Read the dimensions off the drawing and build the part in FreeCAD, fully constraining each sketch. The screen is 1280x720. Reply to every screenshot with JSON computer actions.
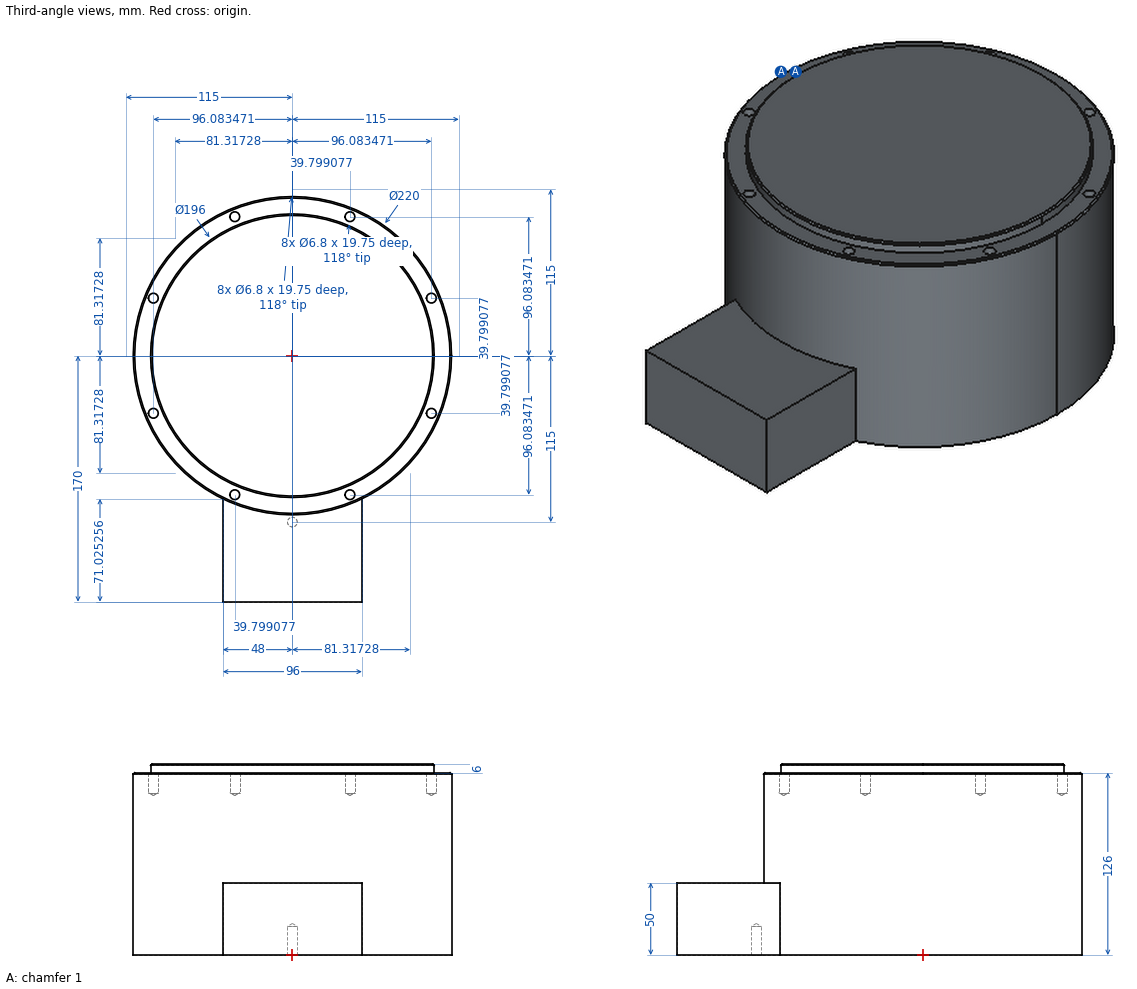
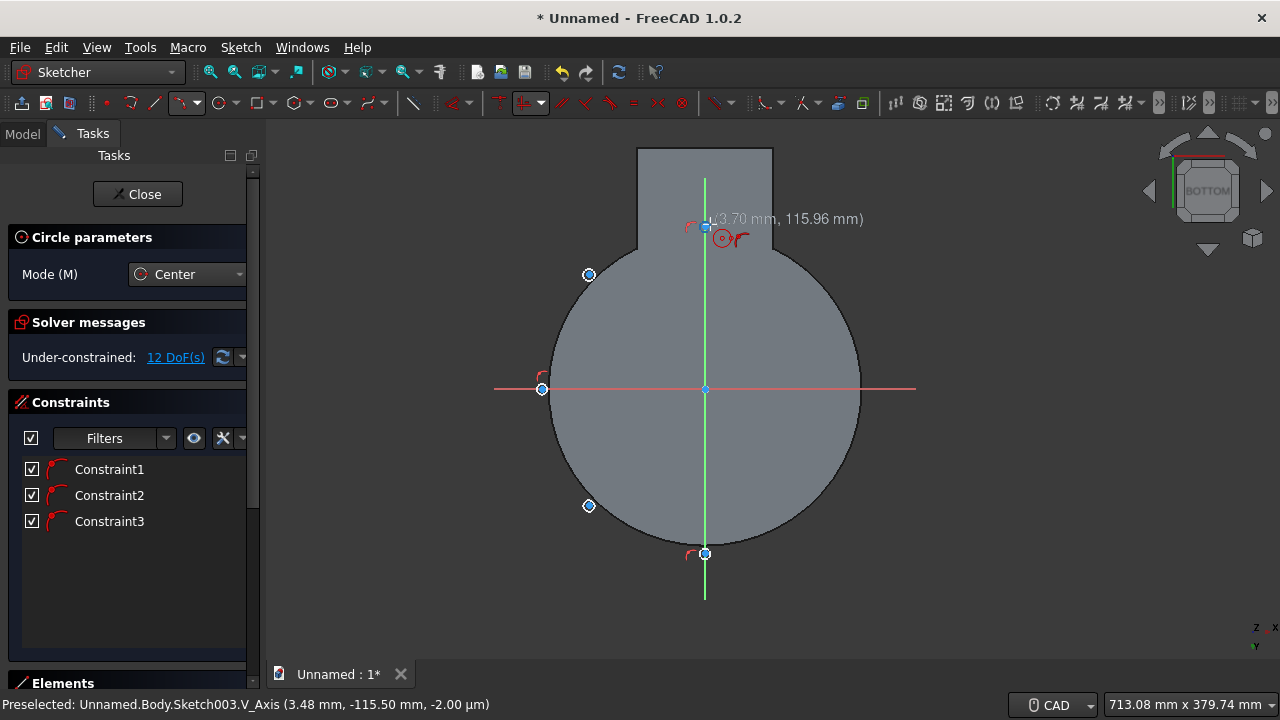
{"action": "scroll", "coordinate": [821, 274], "scroll_direction": "up", "scroll_amount": 8}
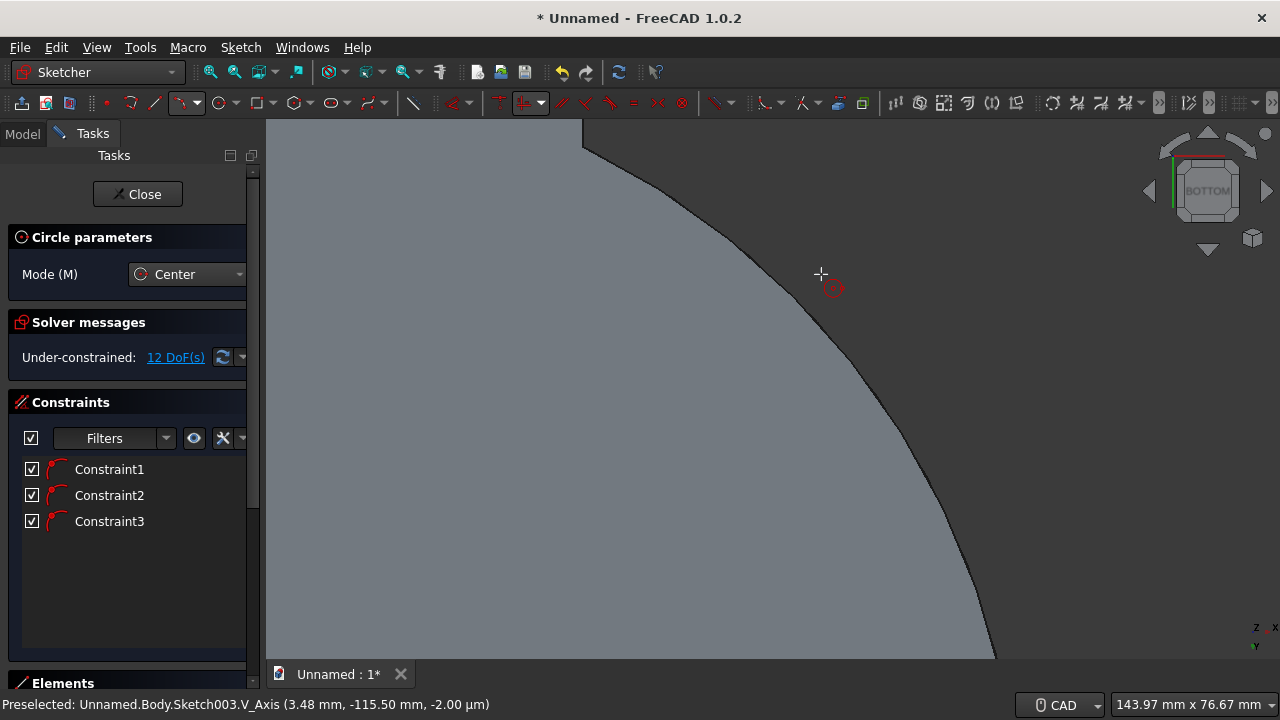
{"action": "scroll", "coordinate": [821, 274], "scroll_direction": "down", "scroll_amount": 8}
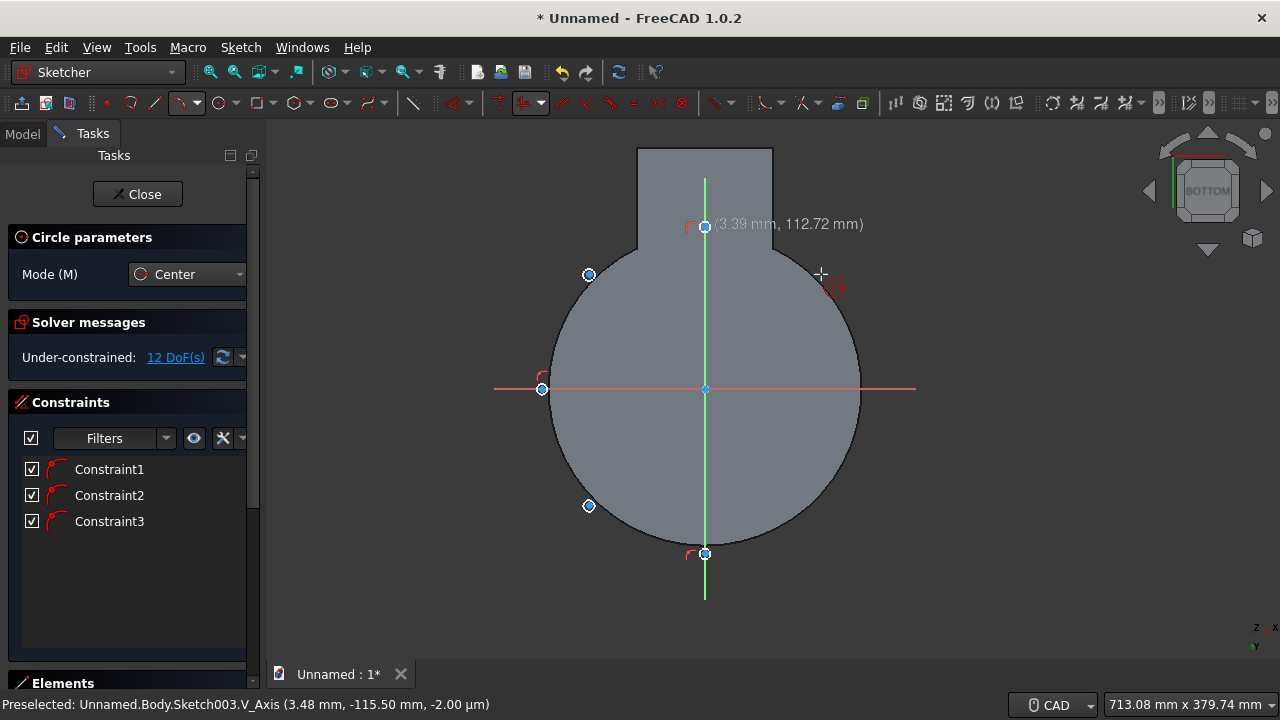
{"action": "left_click", "coordinate": [821, 274]}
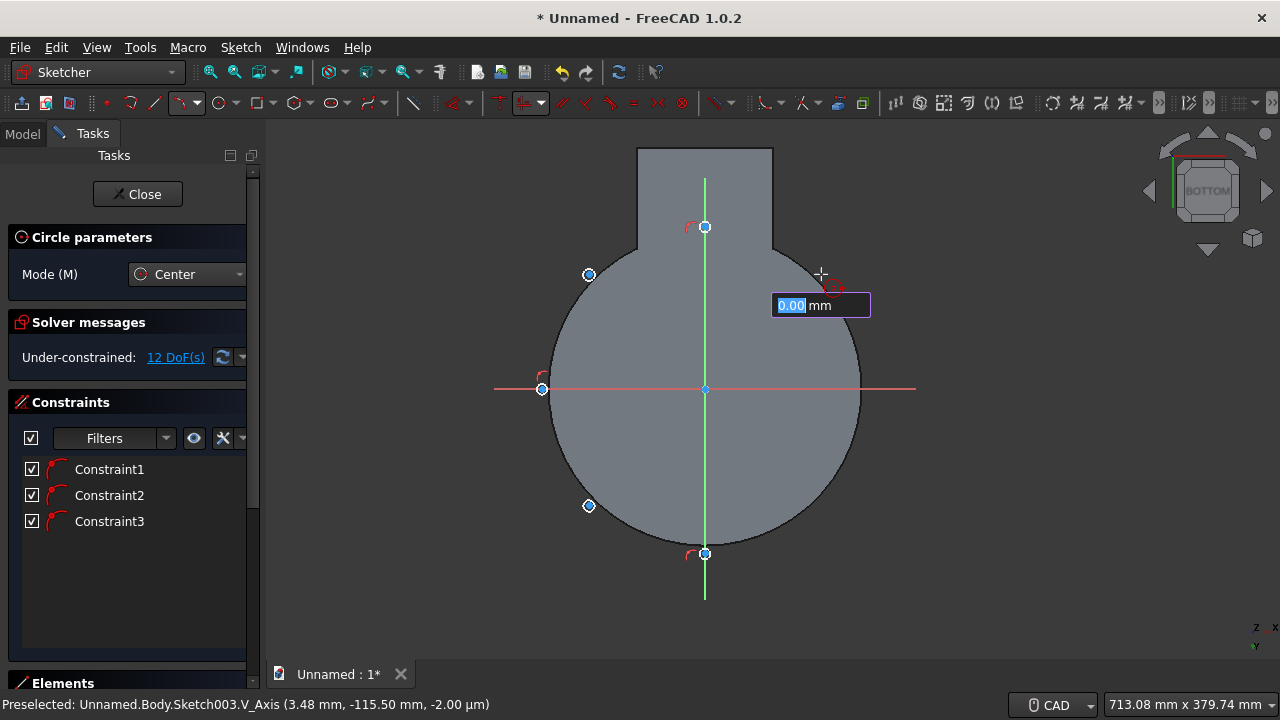
{"action": "scroll", "coordinate": [824, 270], "scroll_direction": "up", "scroll_amount": 6}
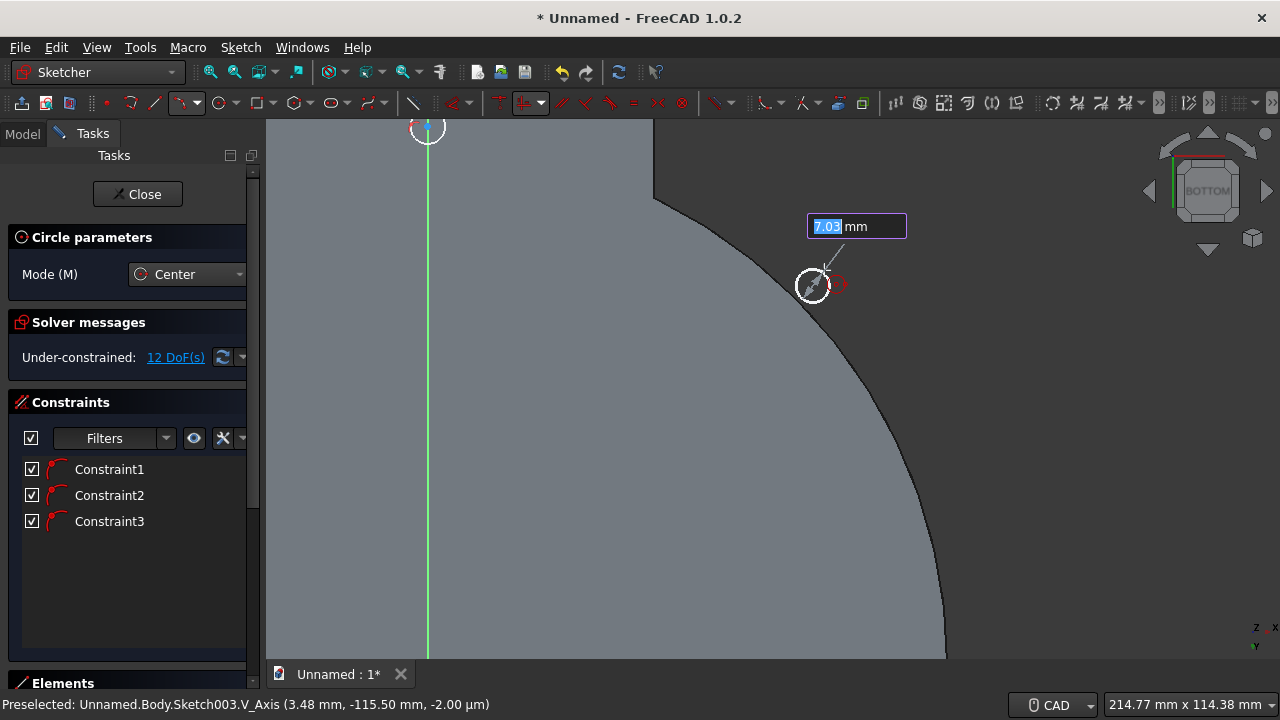
{"action": "left_click", "coordinate": [823, 270]}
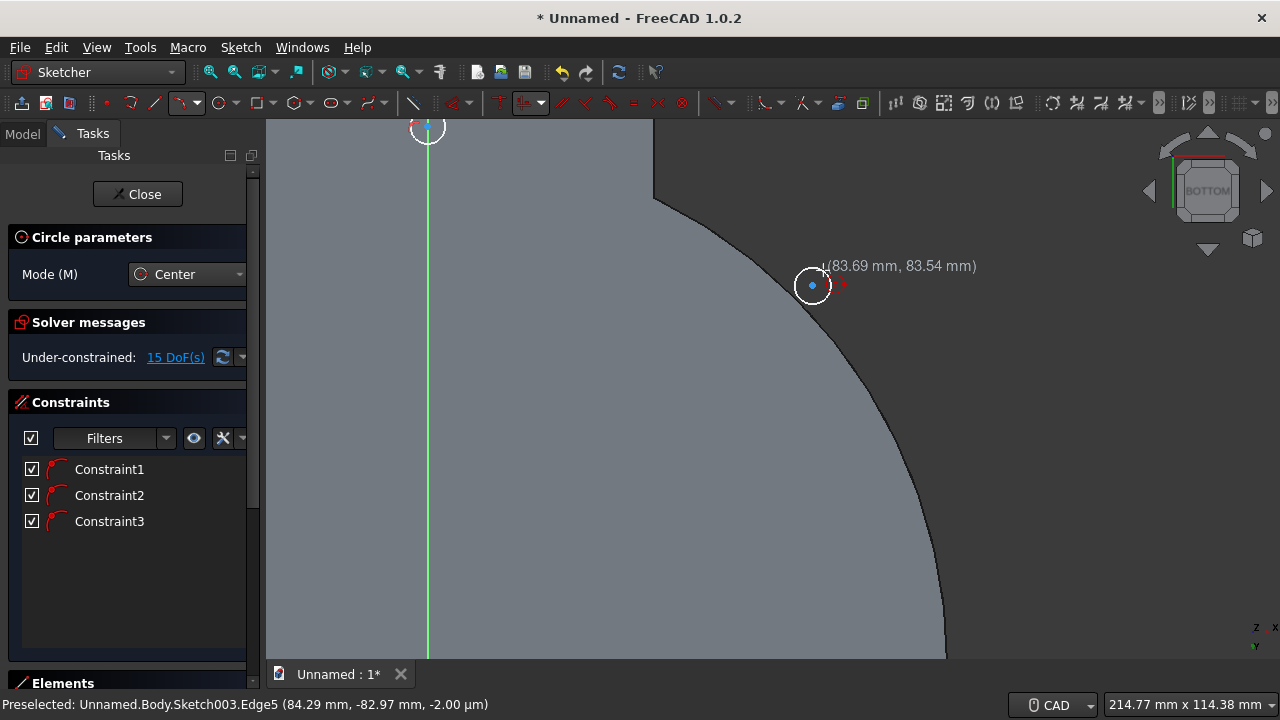
{"action": "scroll", "coordinate": [824, 270], "scroll_direction": "down", "scroll_amount": 6}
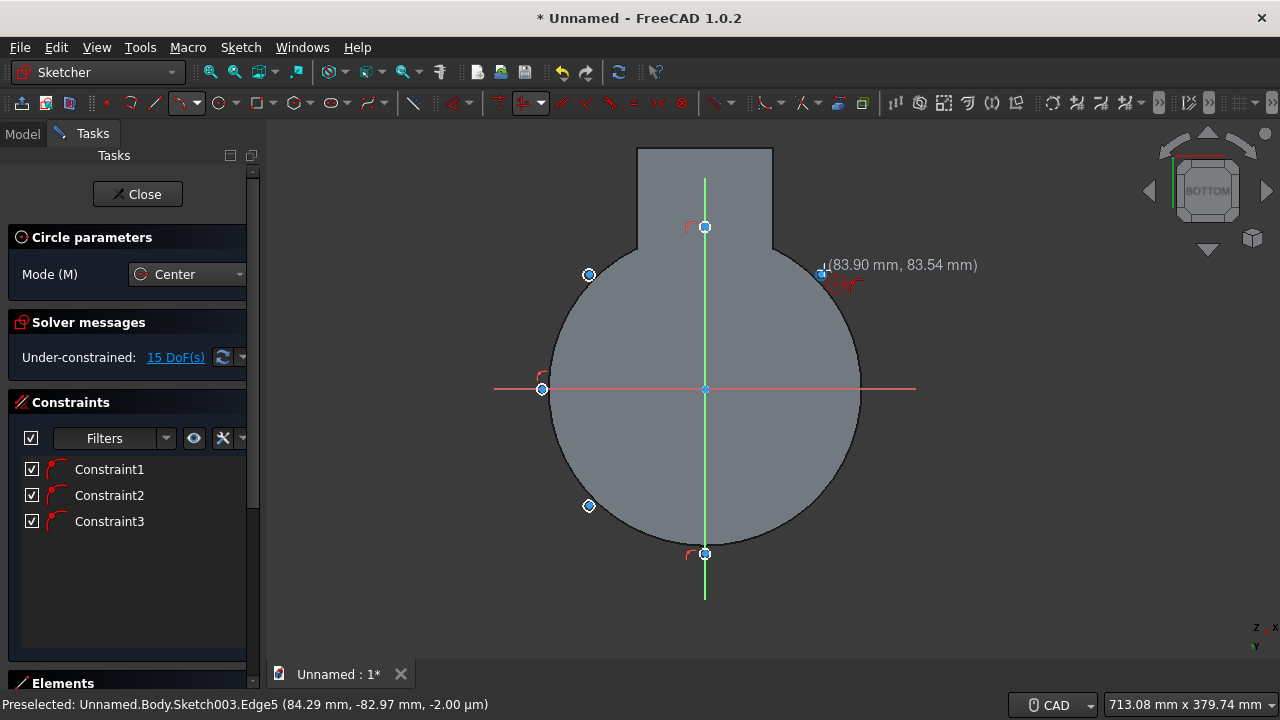
{"action": "scroll", "coordinate": [869, 389], "scroll_direction": "up", "scroll_amount": 8}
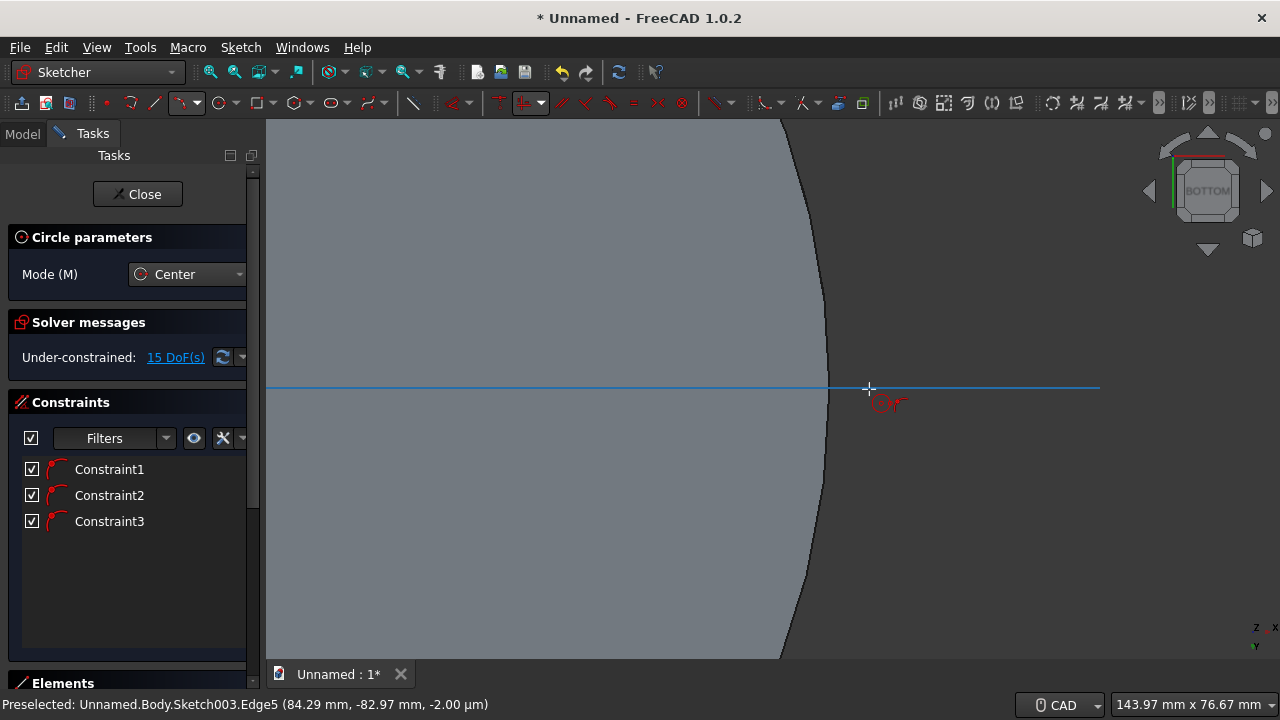
{"action": "scroll", "coordinate": [869, 389], "scroll_direction": "down", "scroll_amount": 8}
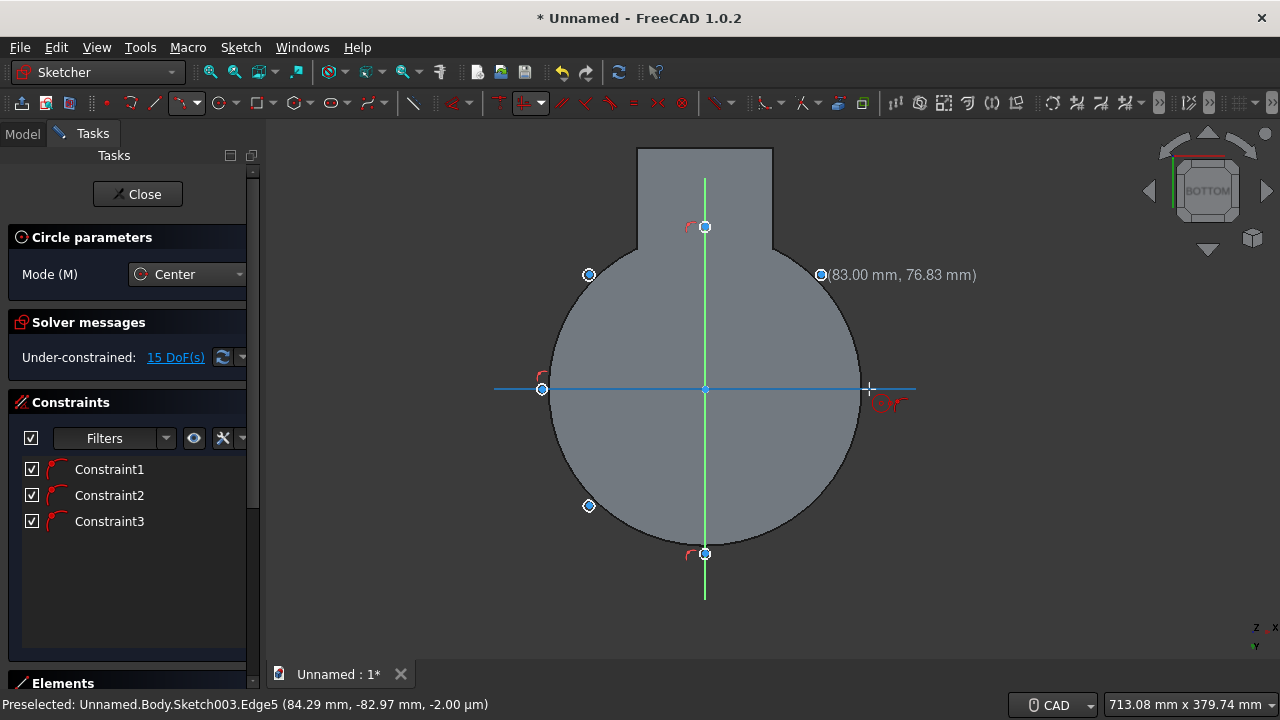
{"action": "left_click", "coordinate": [869, 389]}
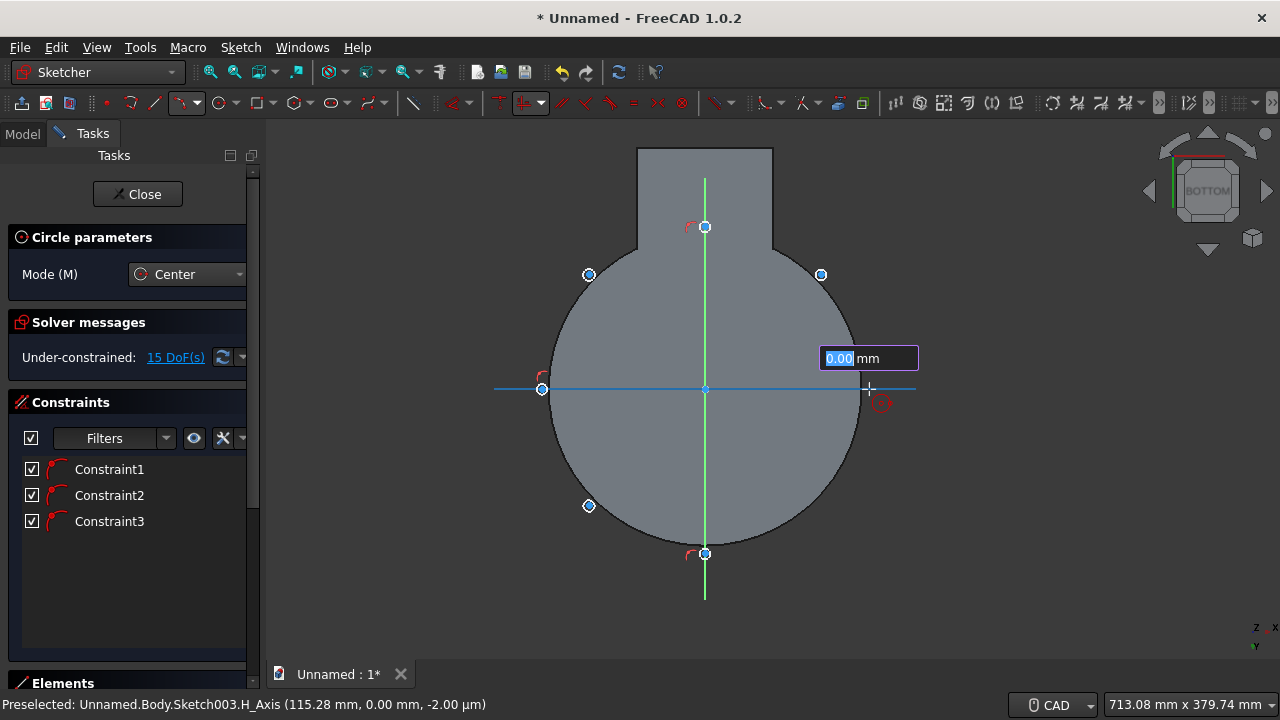
{"action": "scroll", "coordinate": [867, 394], "scroll_direction": "up", "scroll_amount": 7}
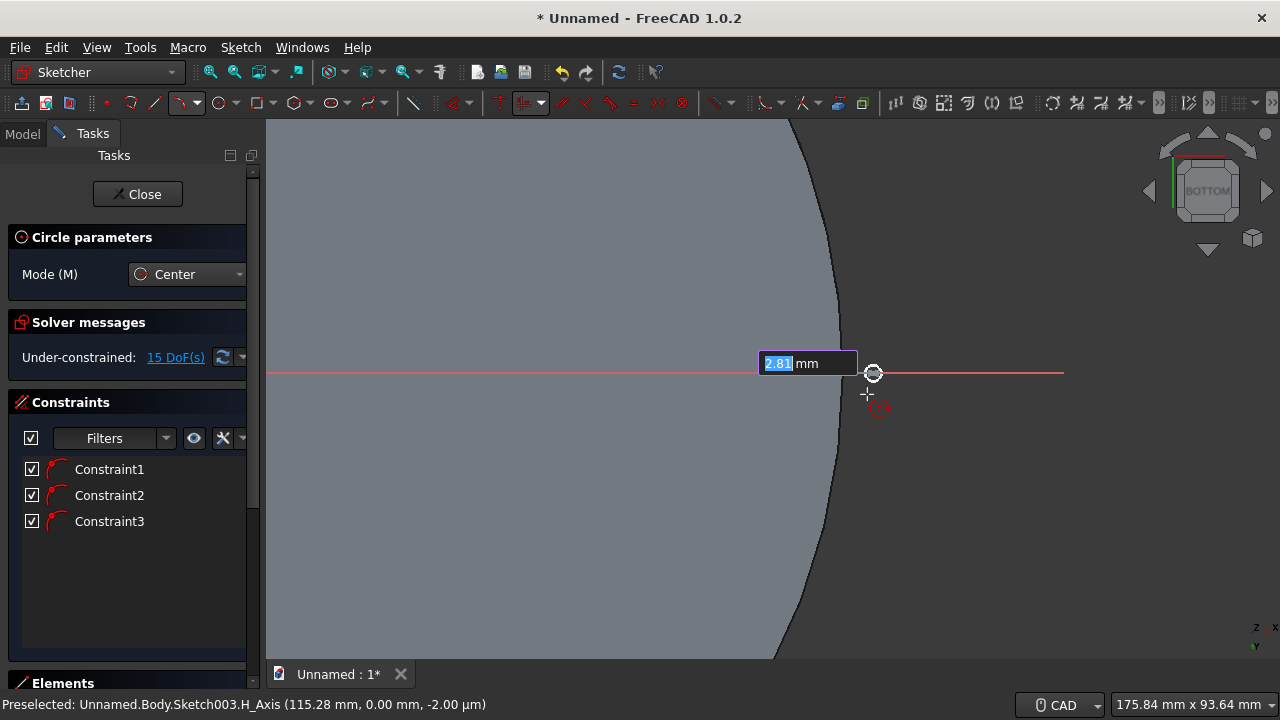
{"action": "left_click", "coordinate": [865, 392]}